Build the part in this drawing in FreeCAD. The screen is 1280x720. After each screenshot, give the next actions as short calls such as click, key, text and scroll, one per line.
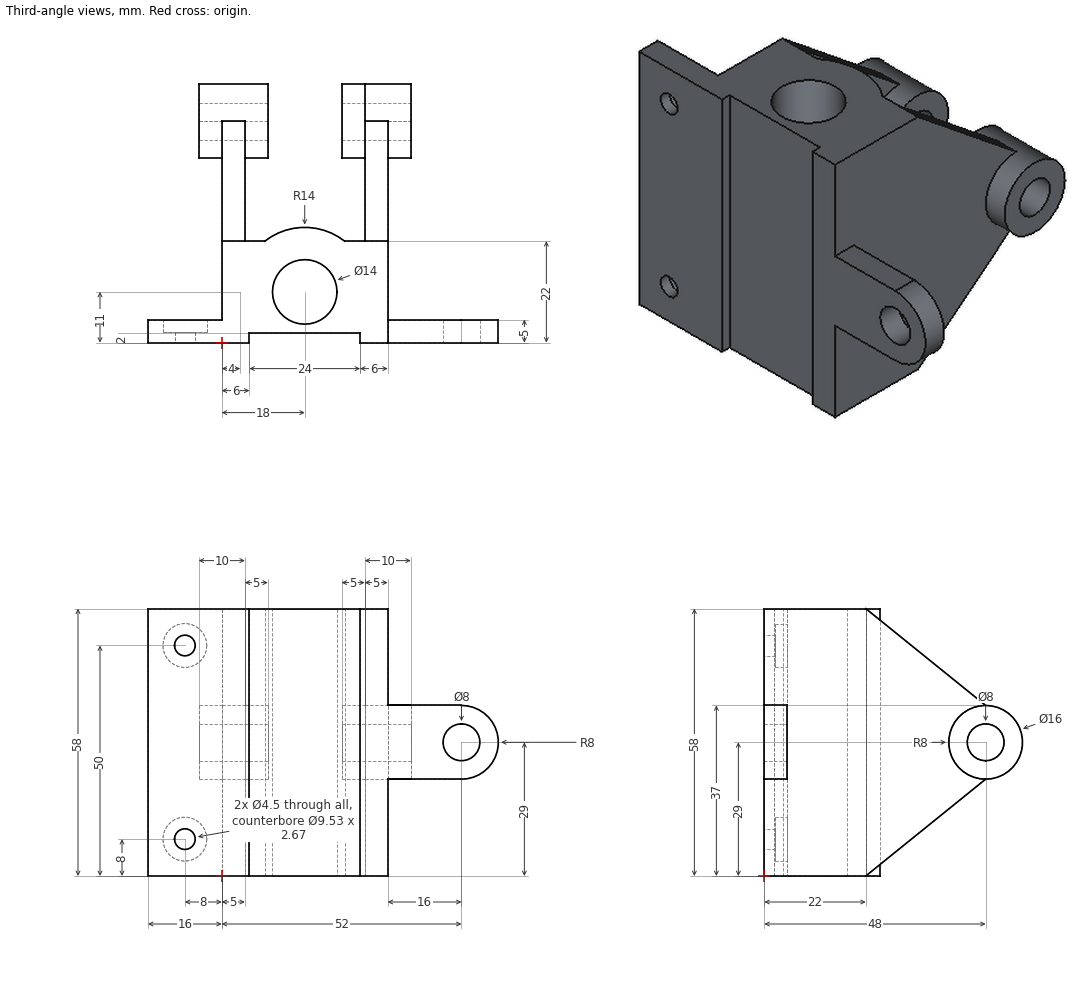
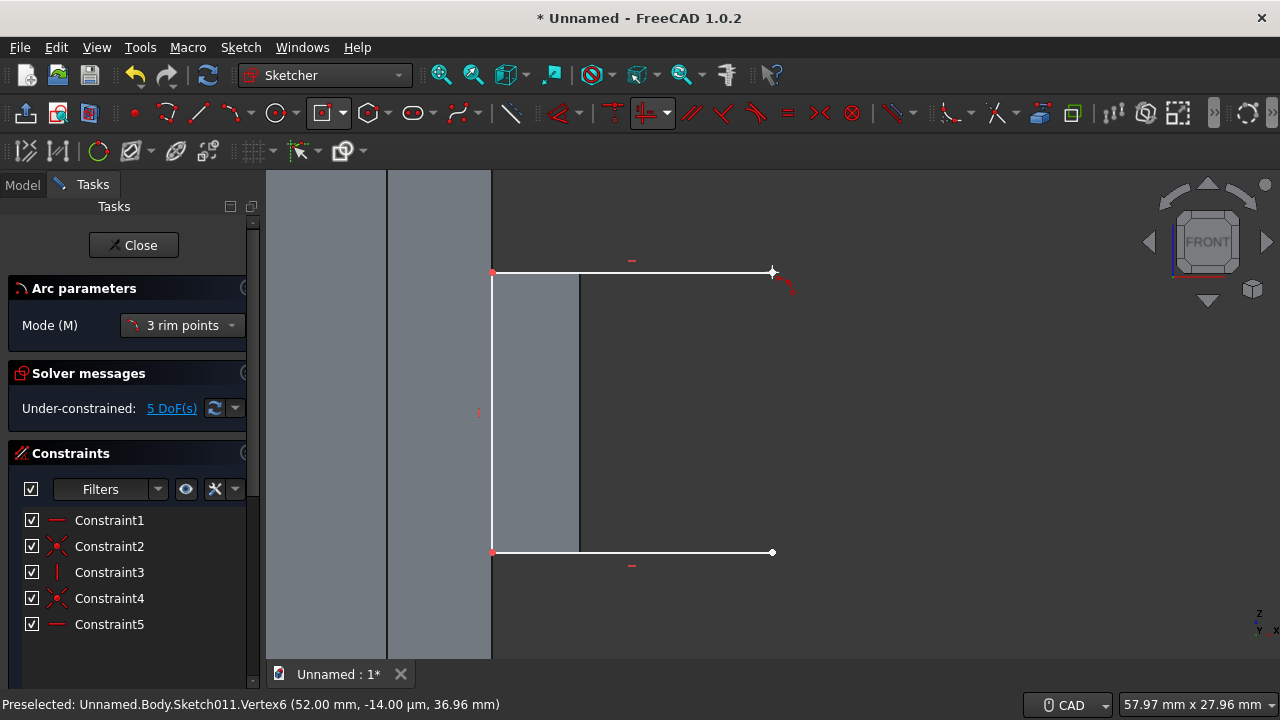
click(772, 273)
click(772, 553)
click(912, 412)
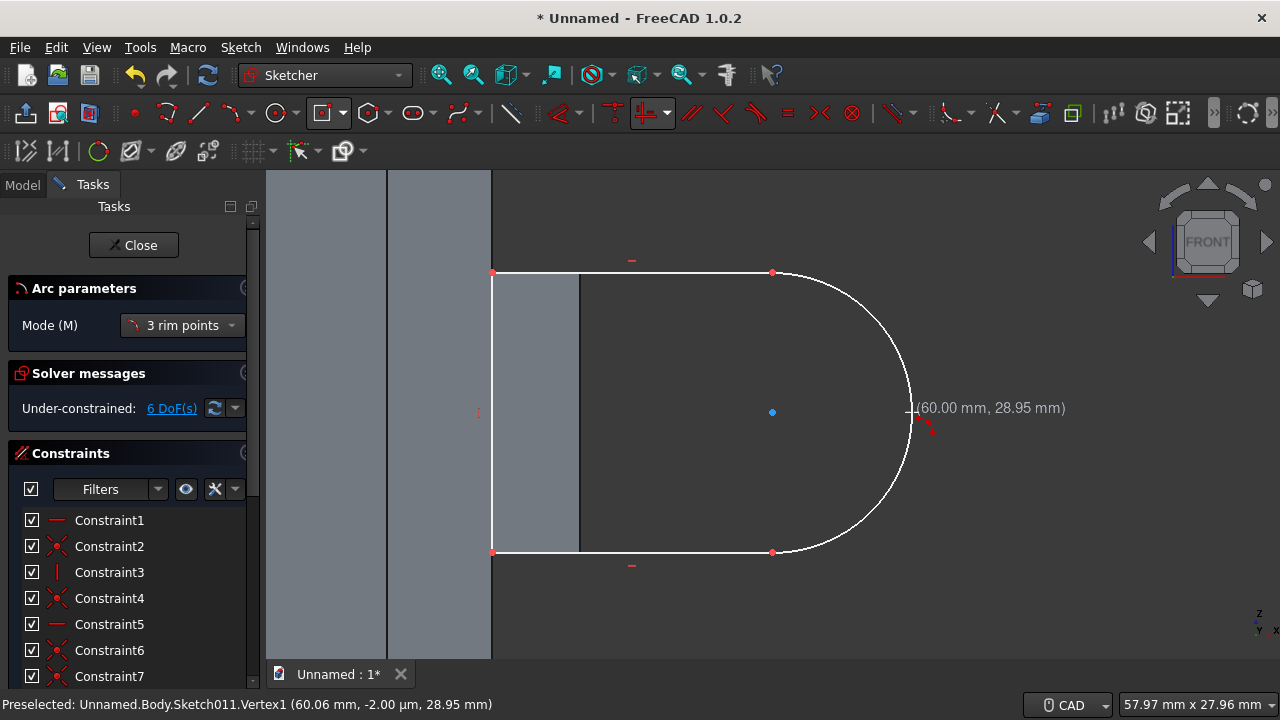
key(g)
key(c)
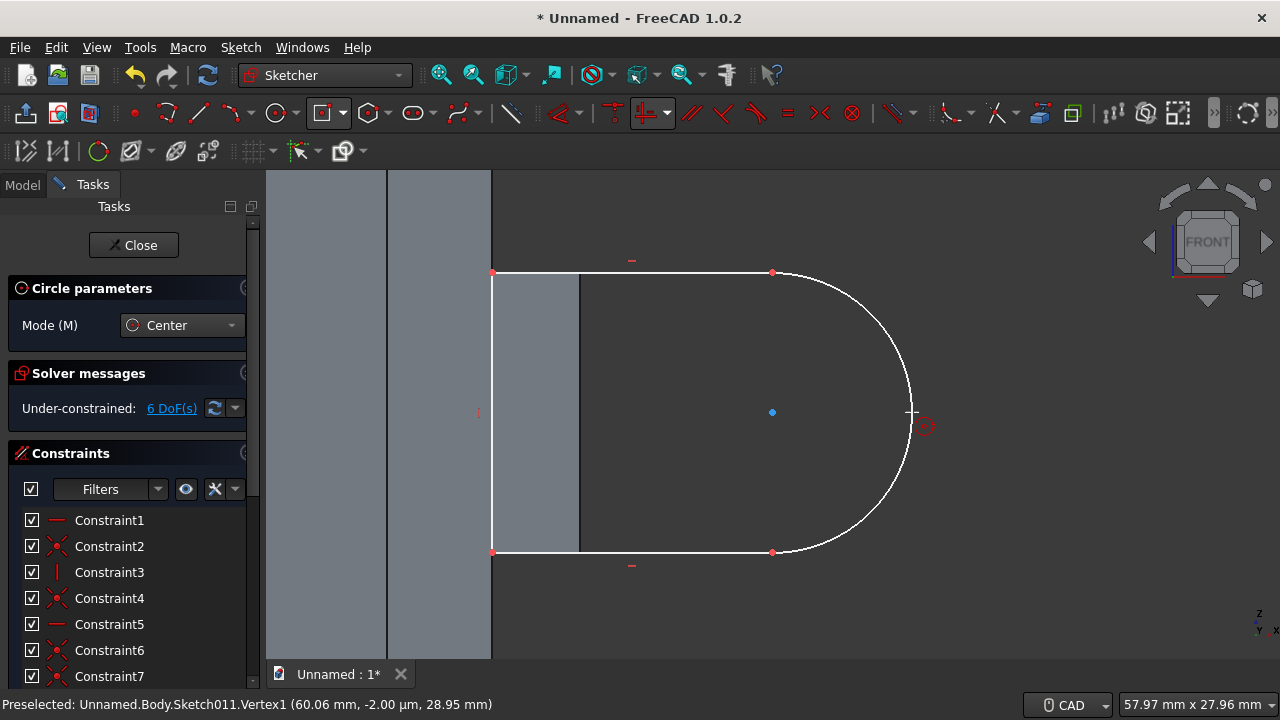
click(772, 412)
move(821, 363)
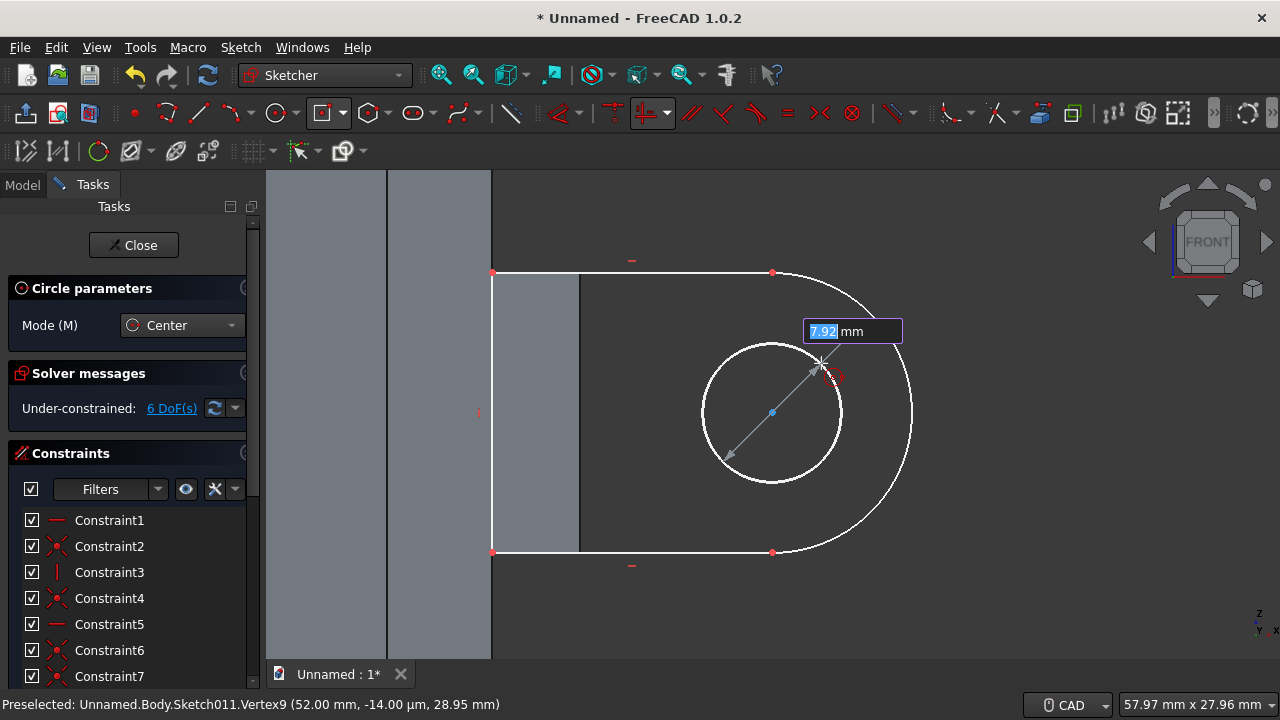
text(8)
key(Return)
key(Escape)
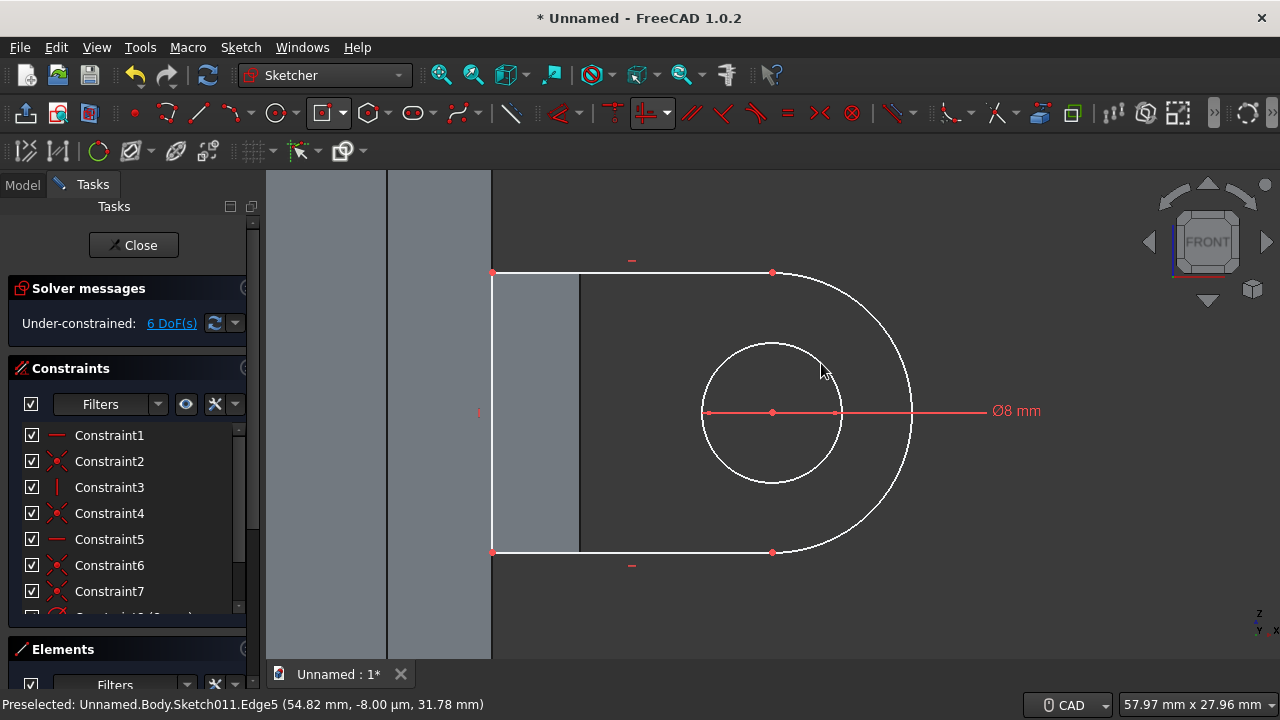
click(688, 553)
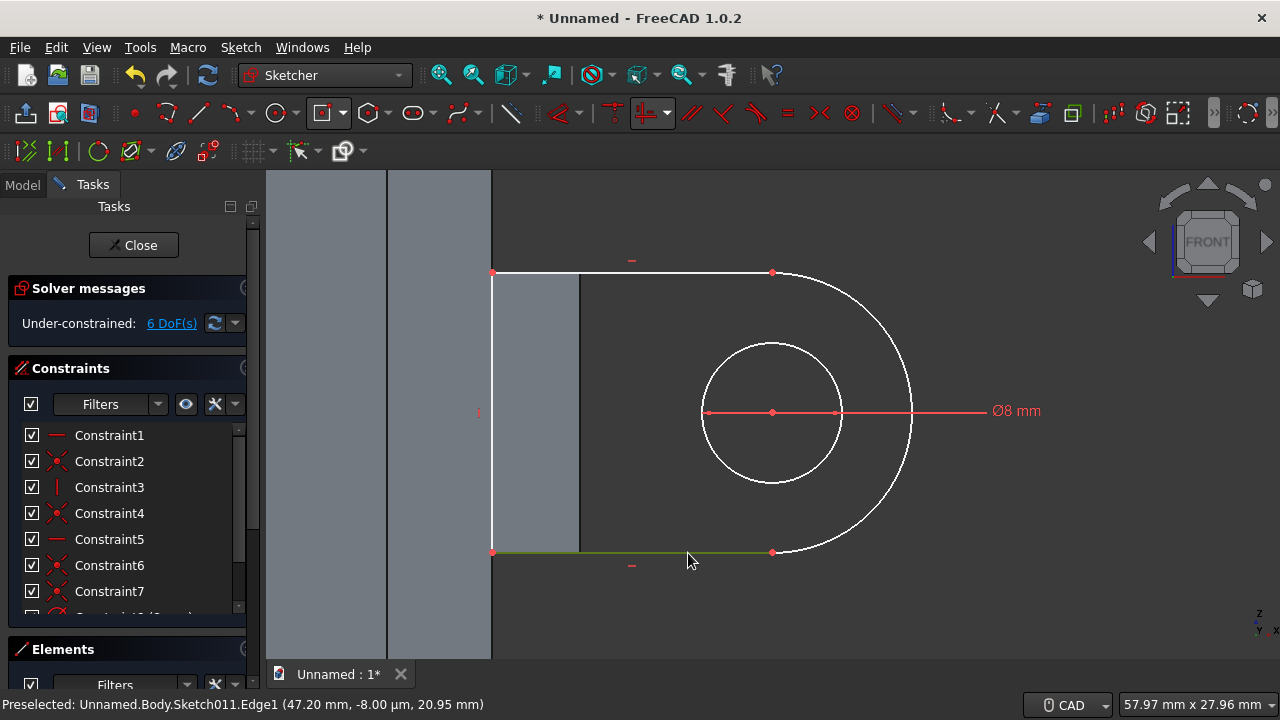
click(885, 495)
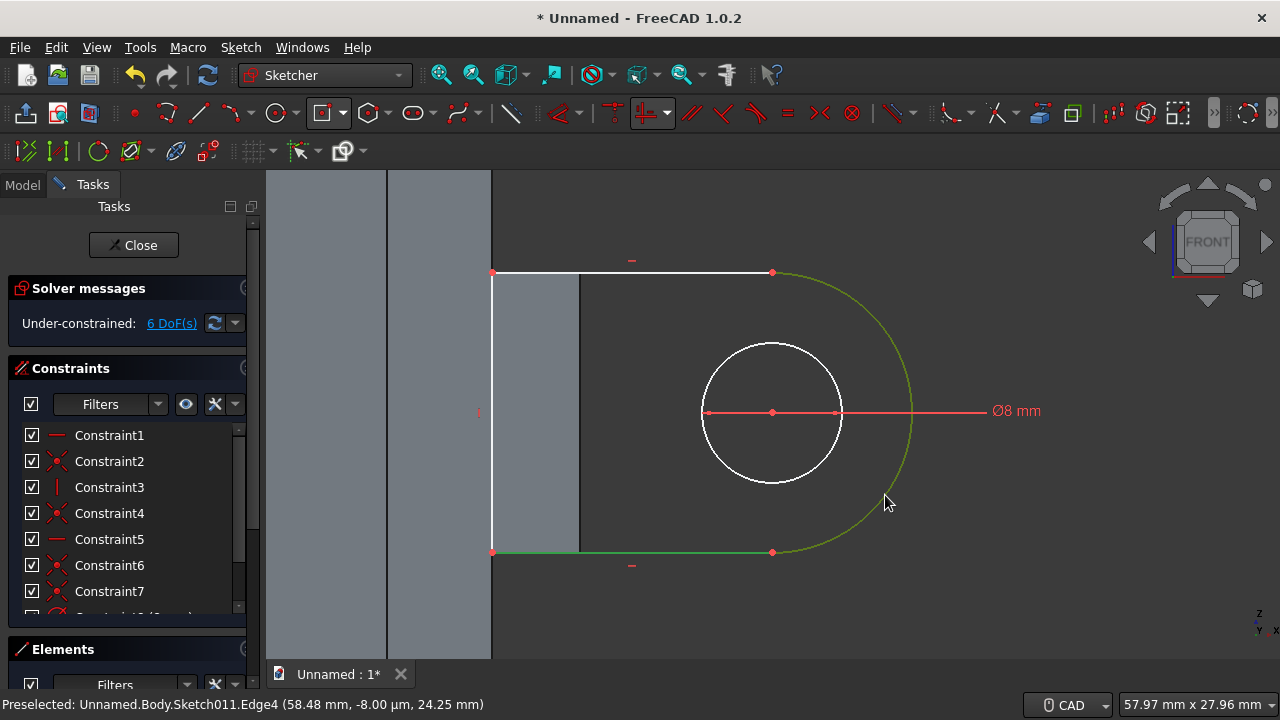
key(t)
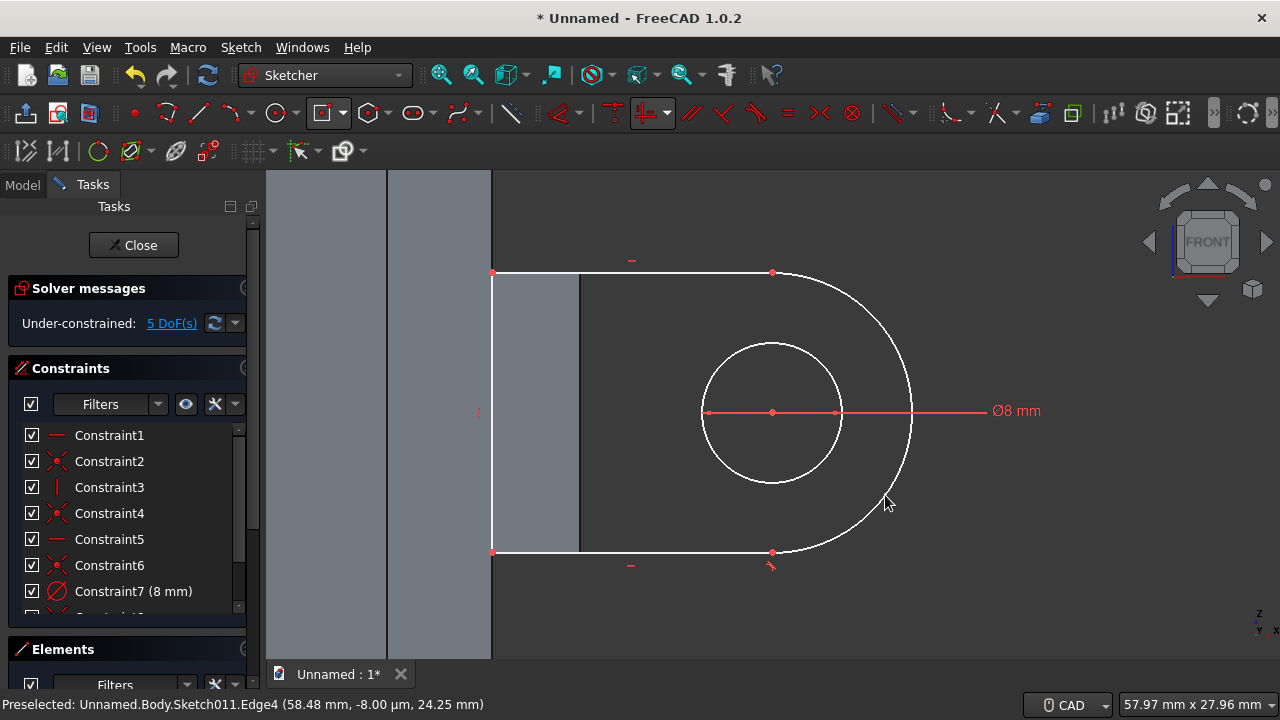
click(576, 273)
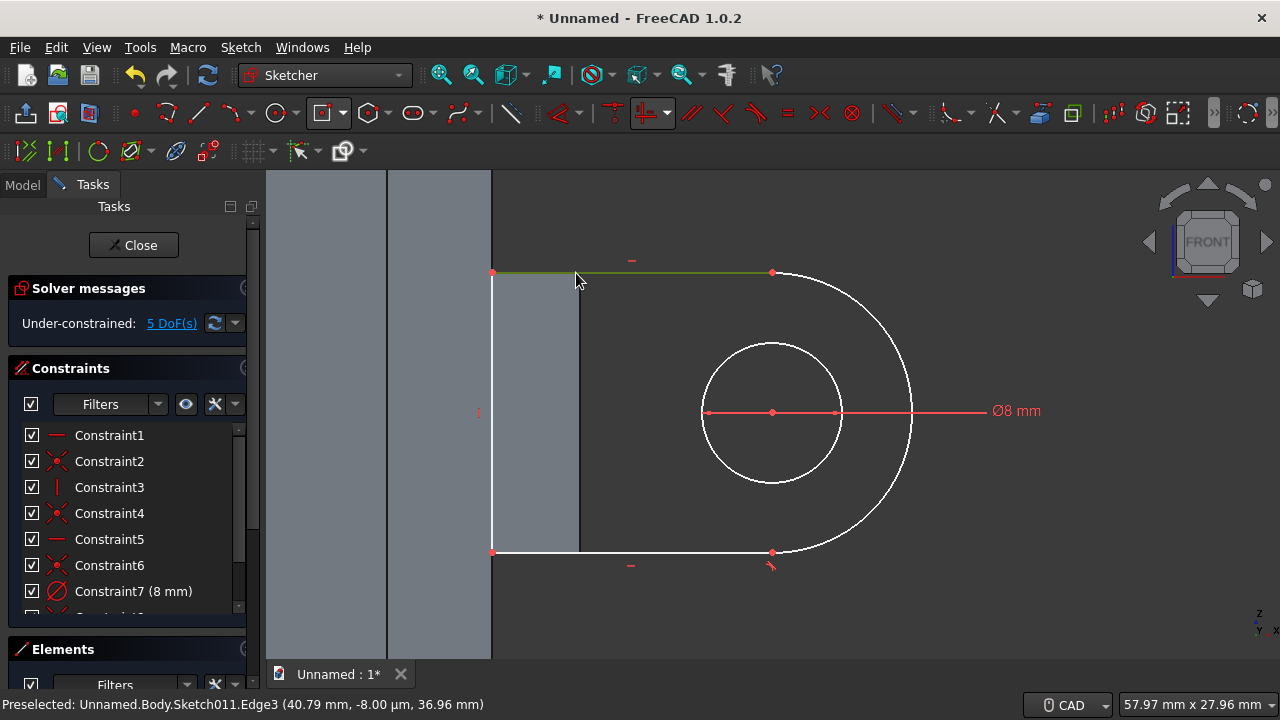
click(885, 495)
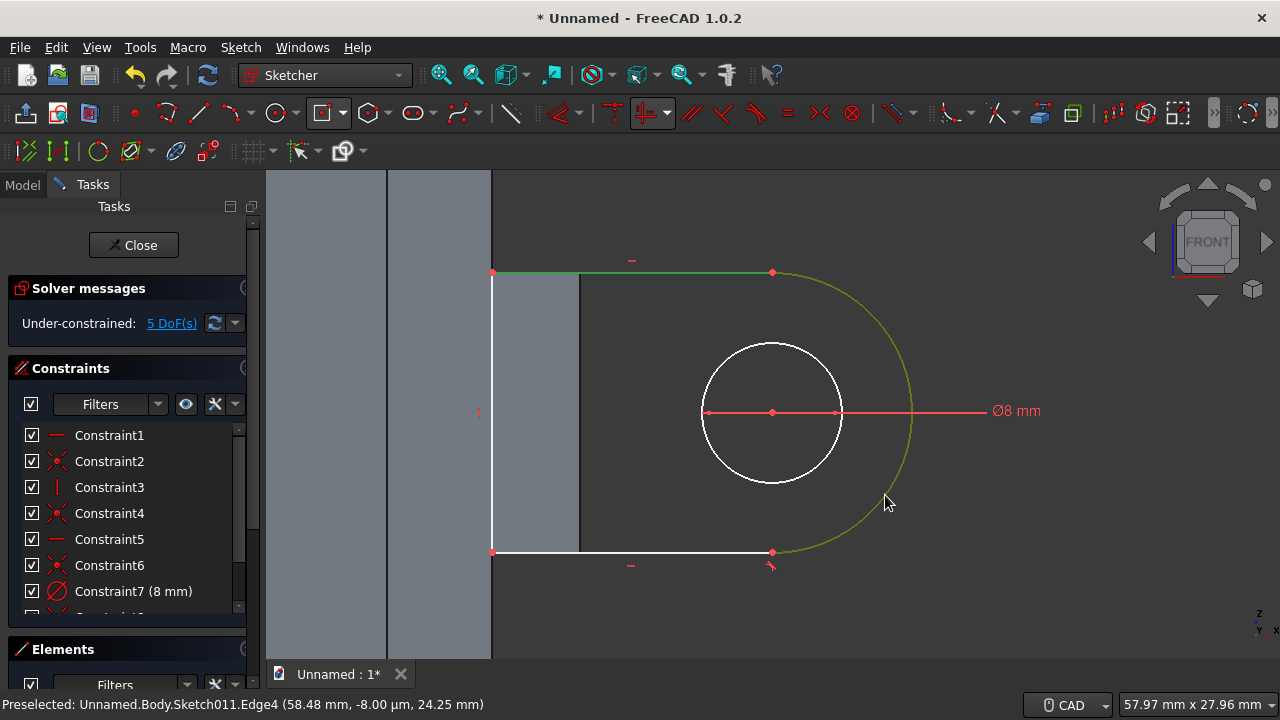
key(t)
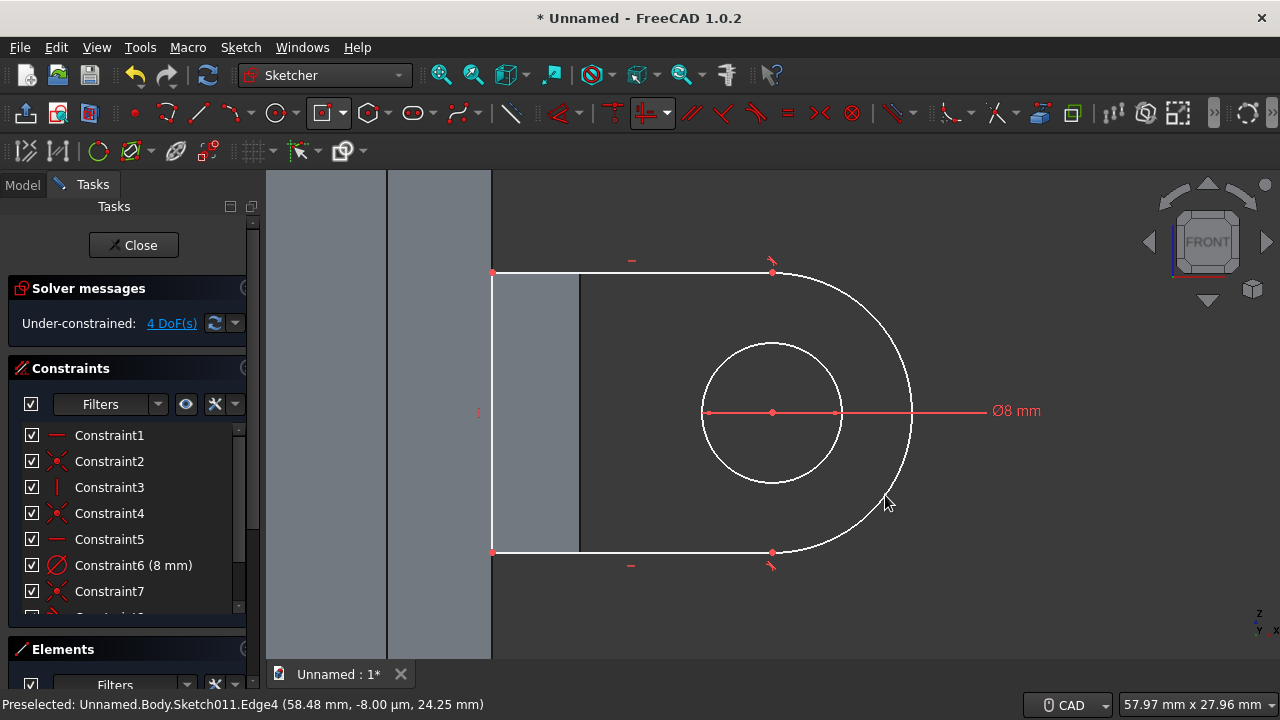
click(558, 114)